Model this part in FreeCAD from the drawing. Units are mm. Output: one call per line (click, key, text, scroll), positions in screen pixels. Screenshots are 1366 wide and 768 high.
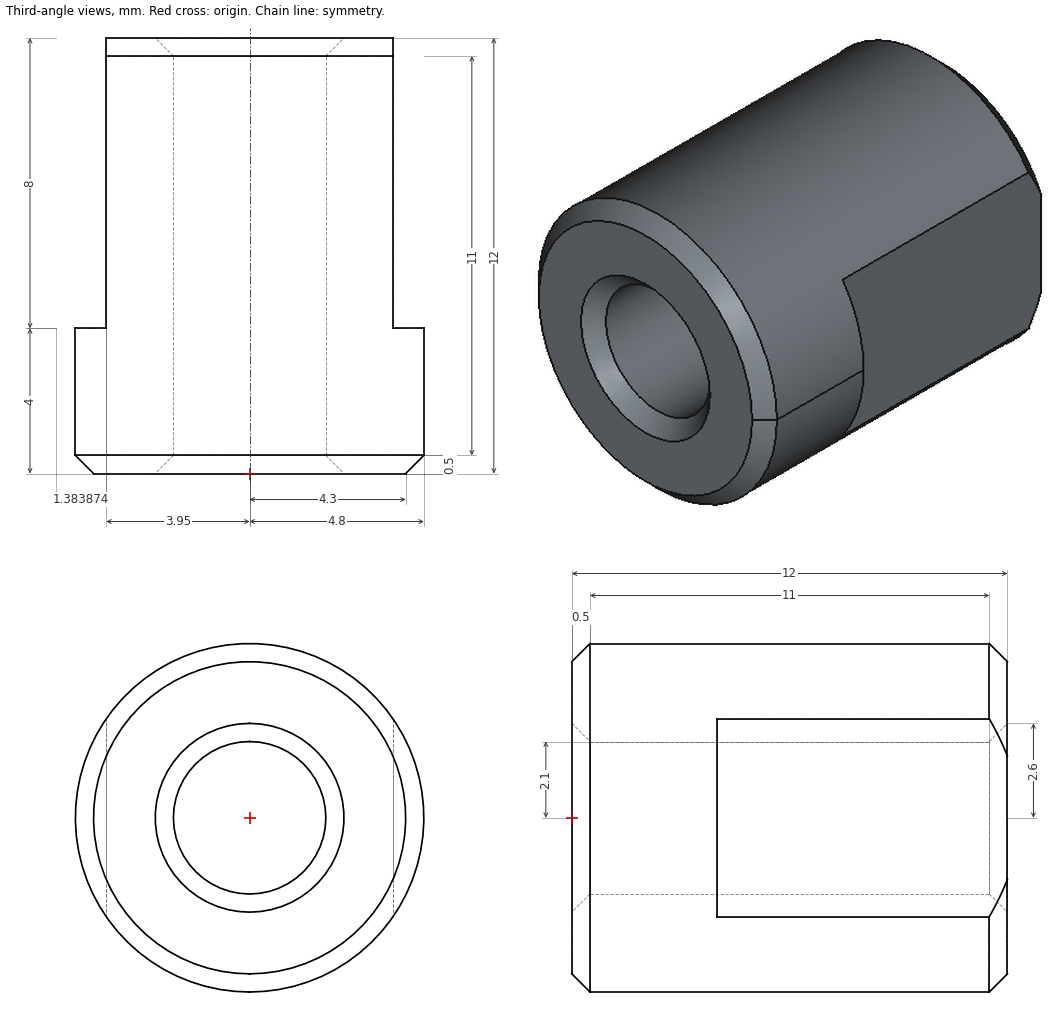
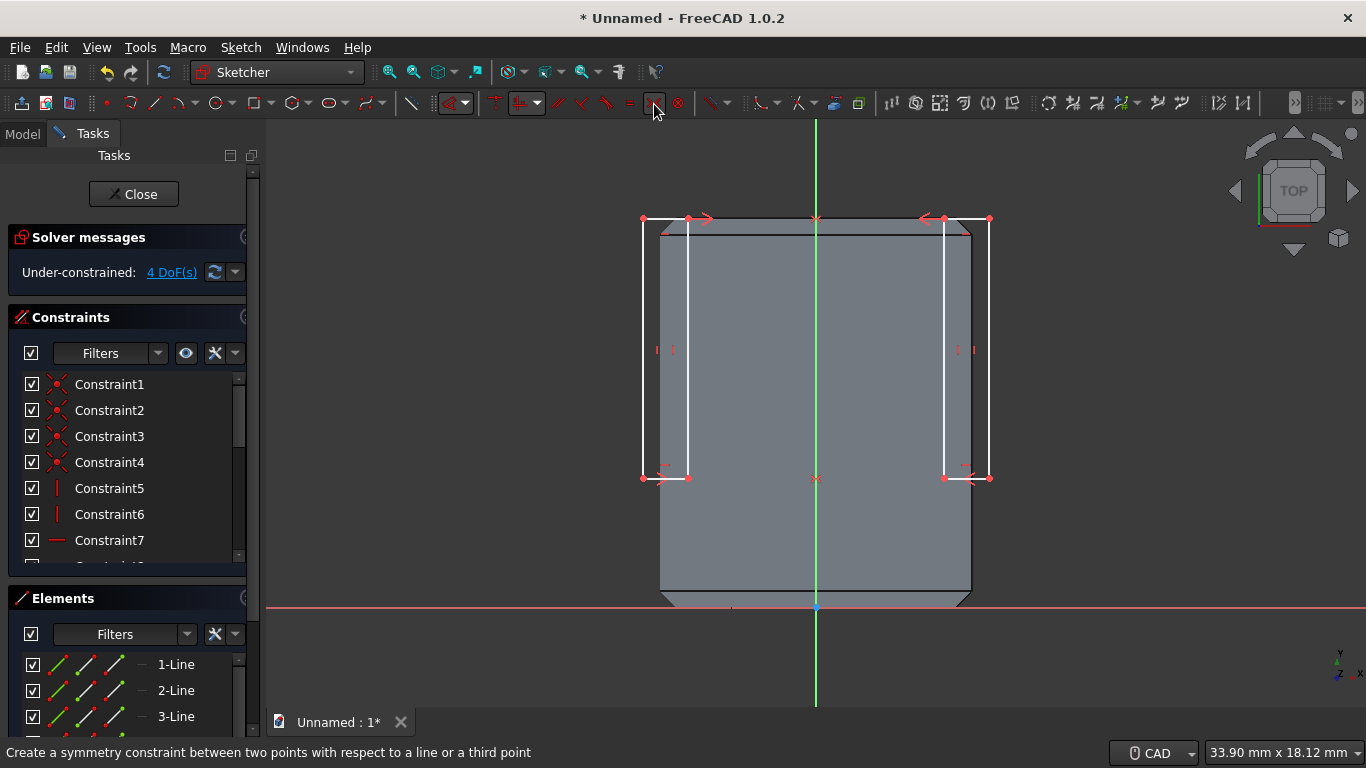
click(643, 297)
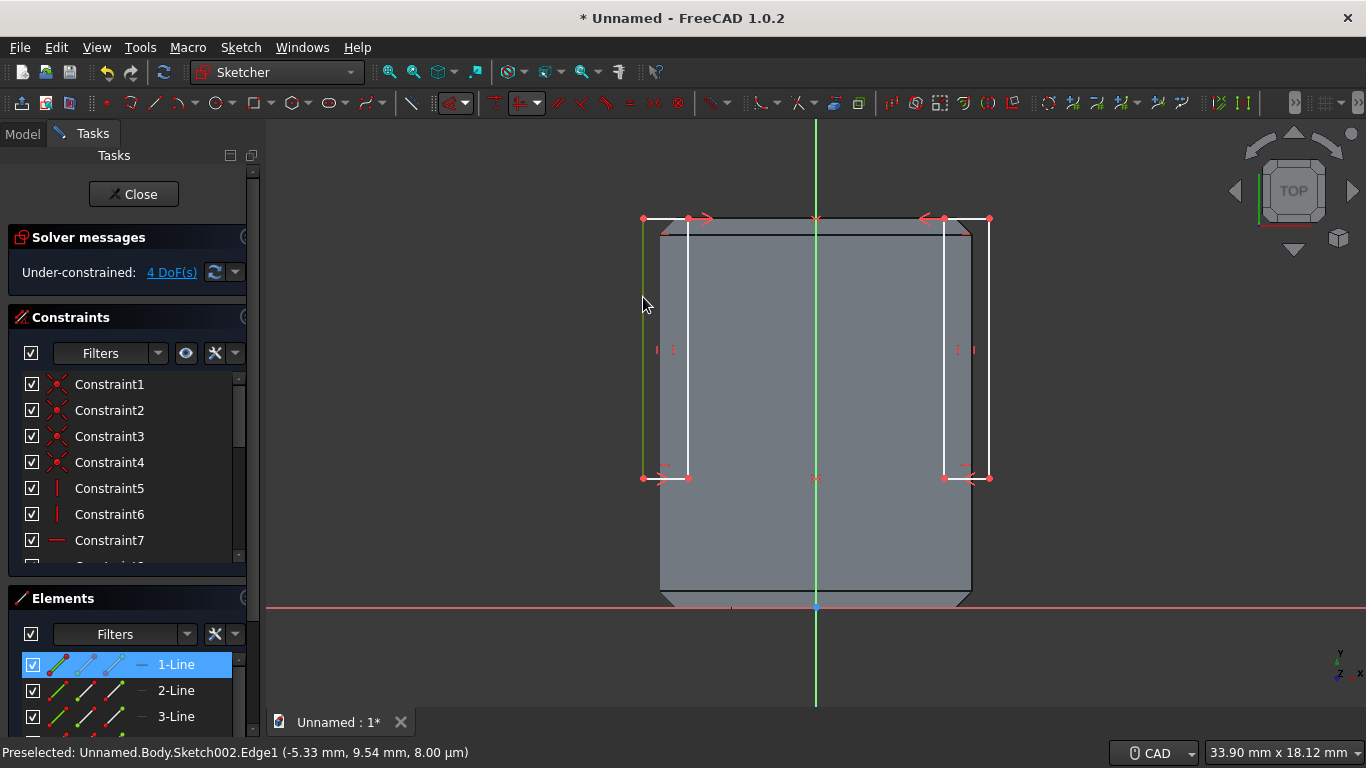
key(i)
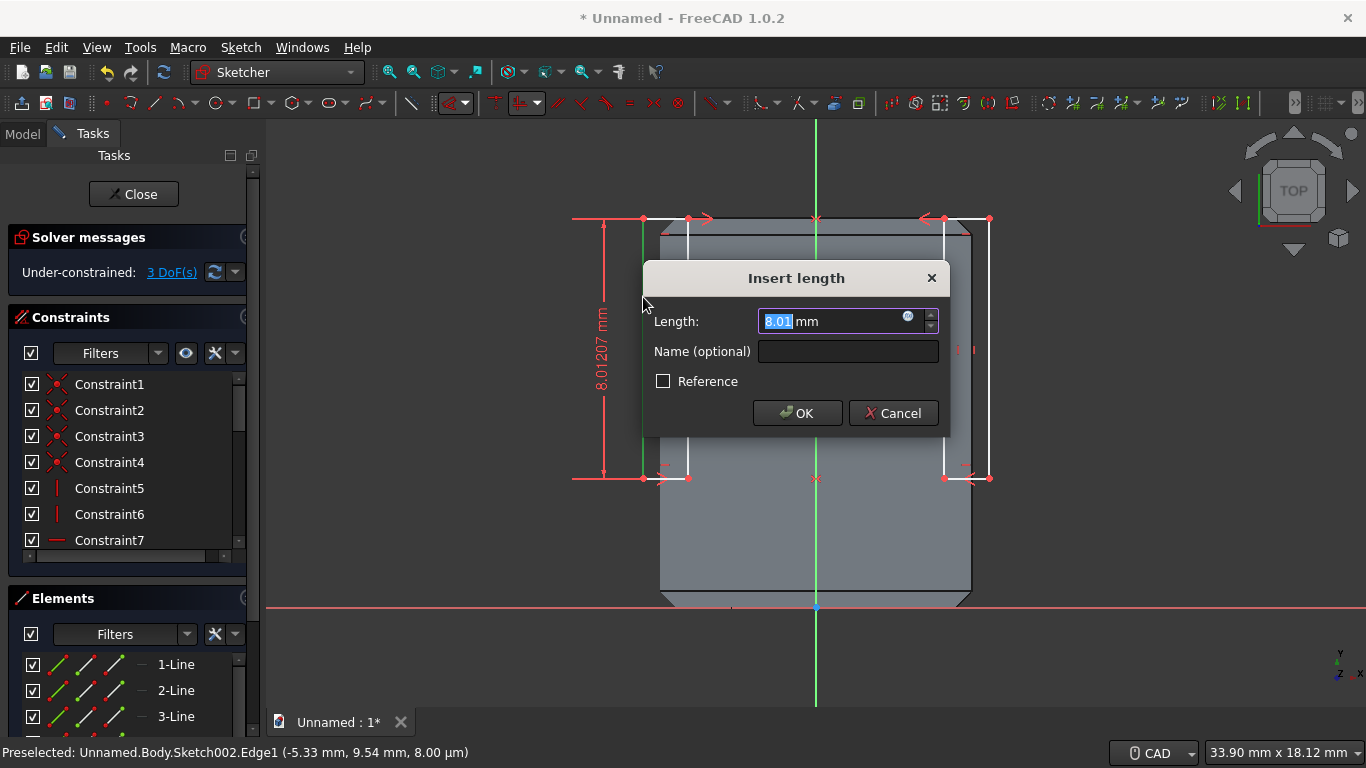
text(8)
key(Return)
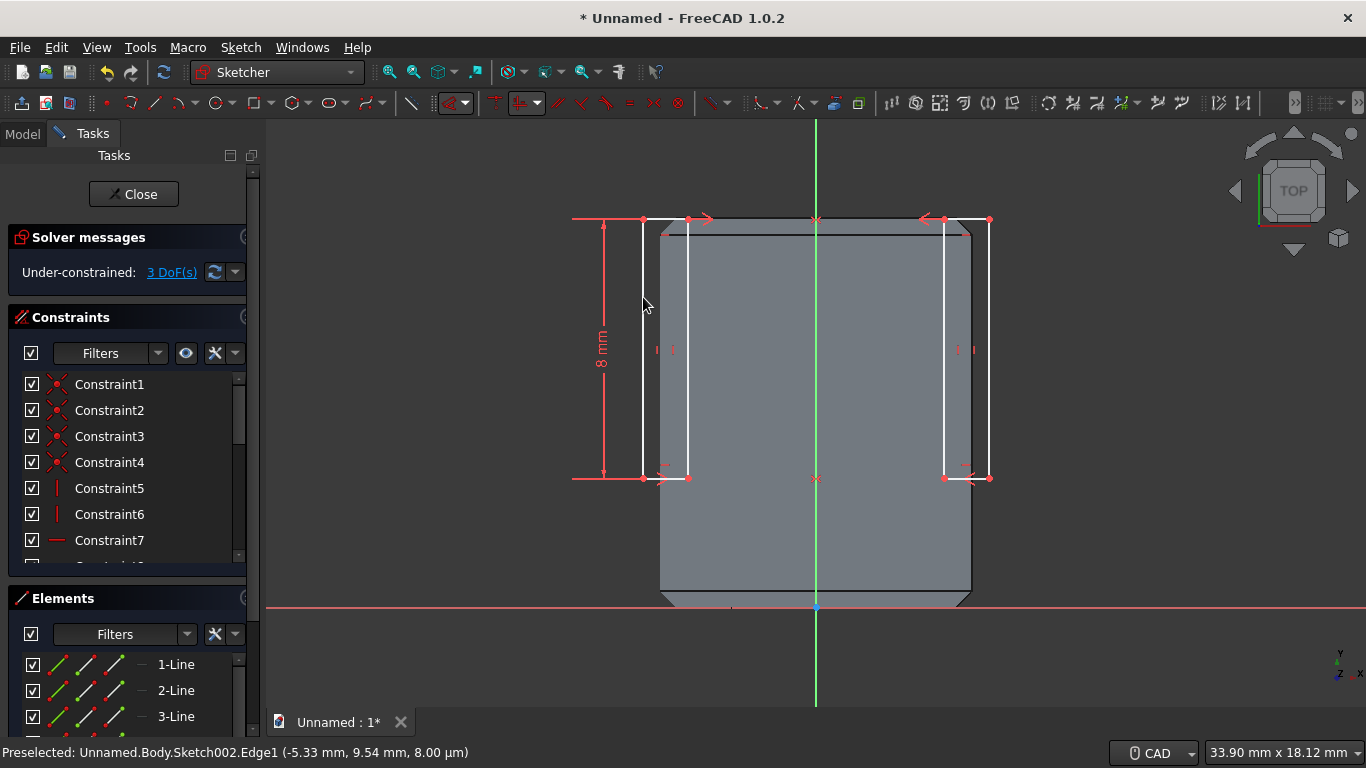
click(643, 479)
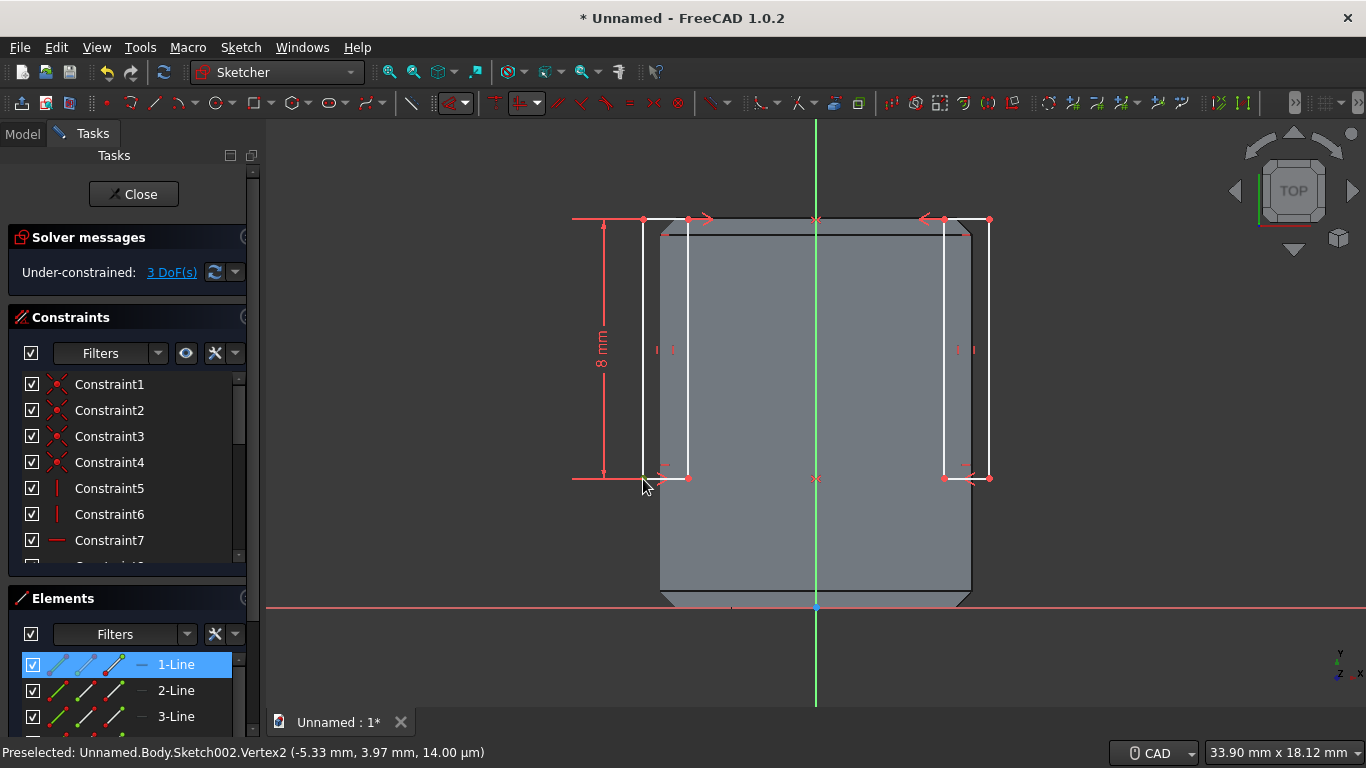
click(468, 104)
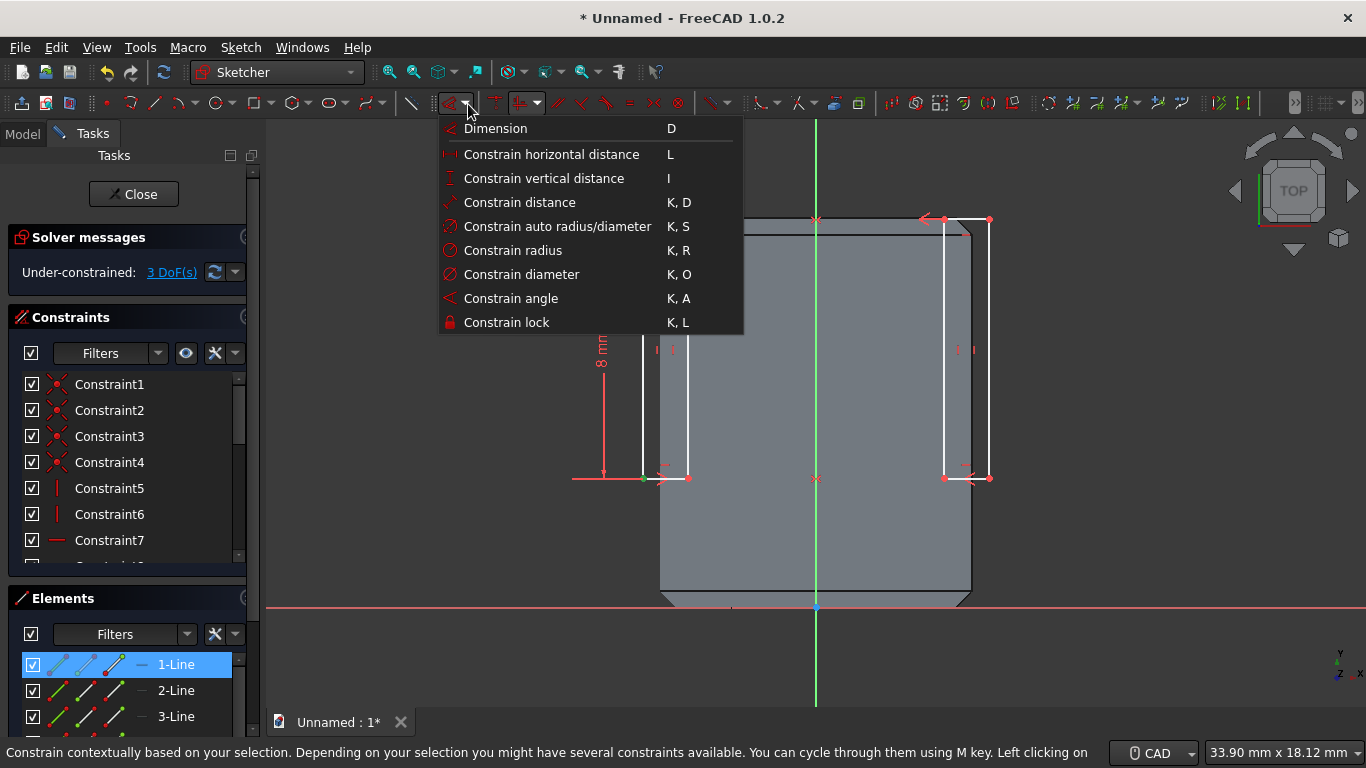
click(591, 178)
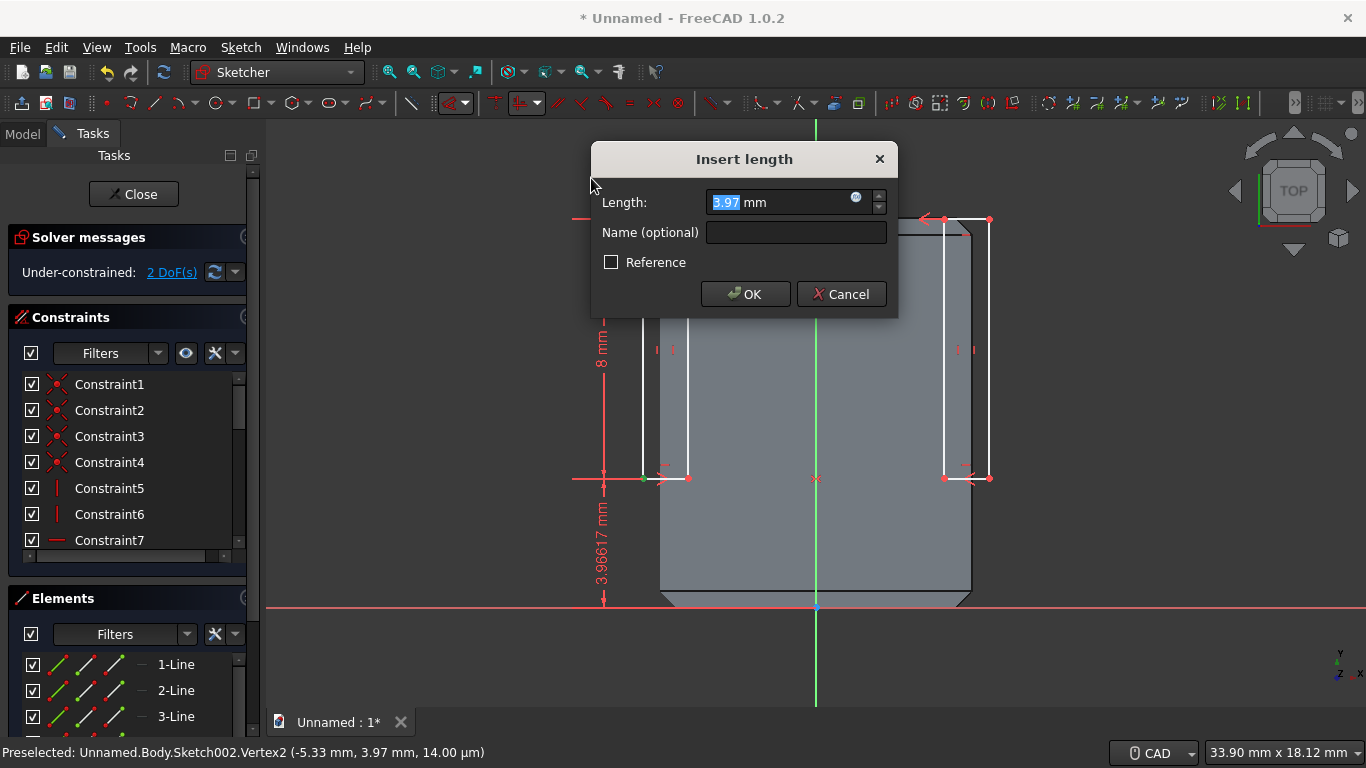
text(4)
key(Return)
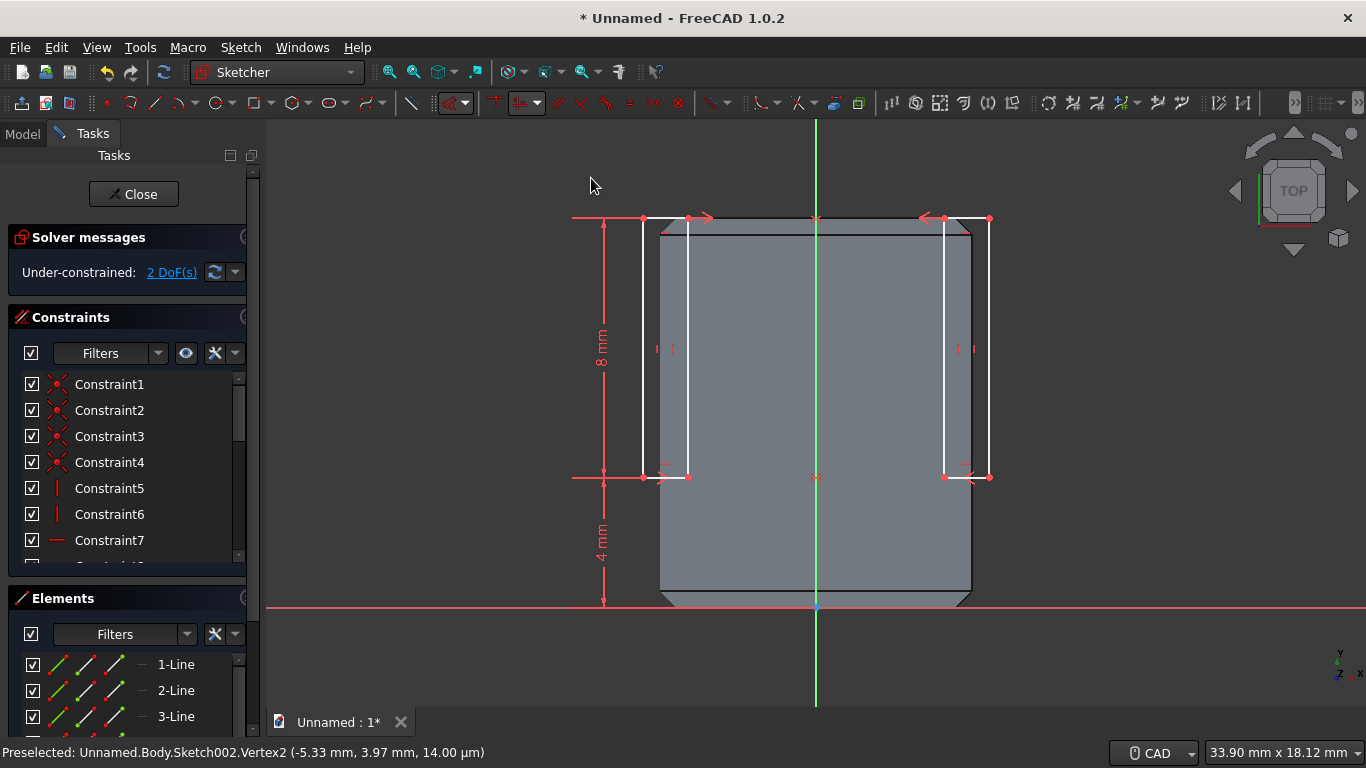
click(688, 478)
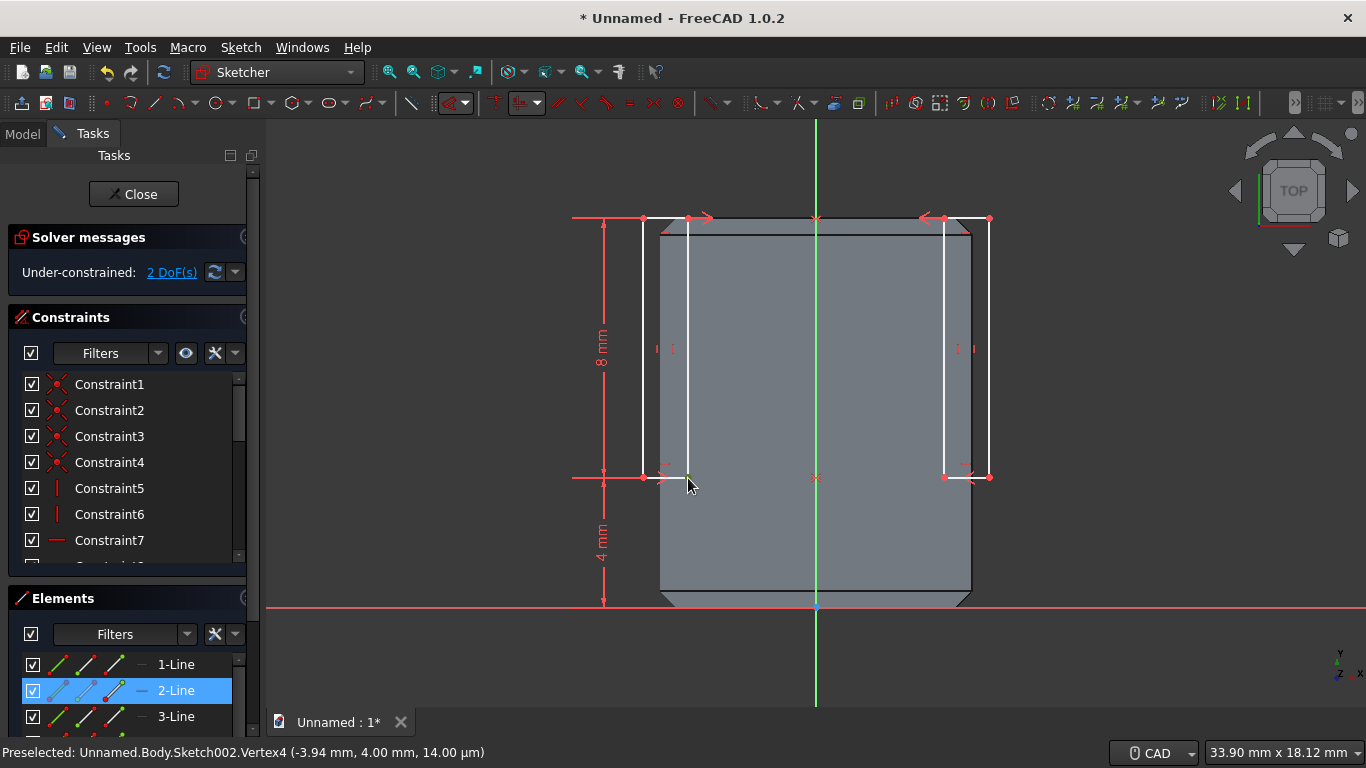
click(468, 104)